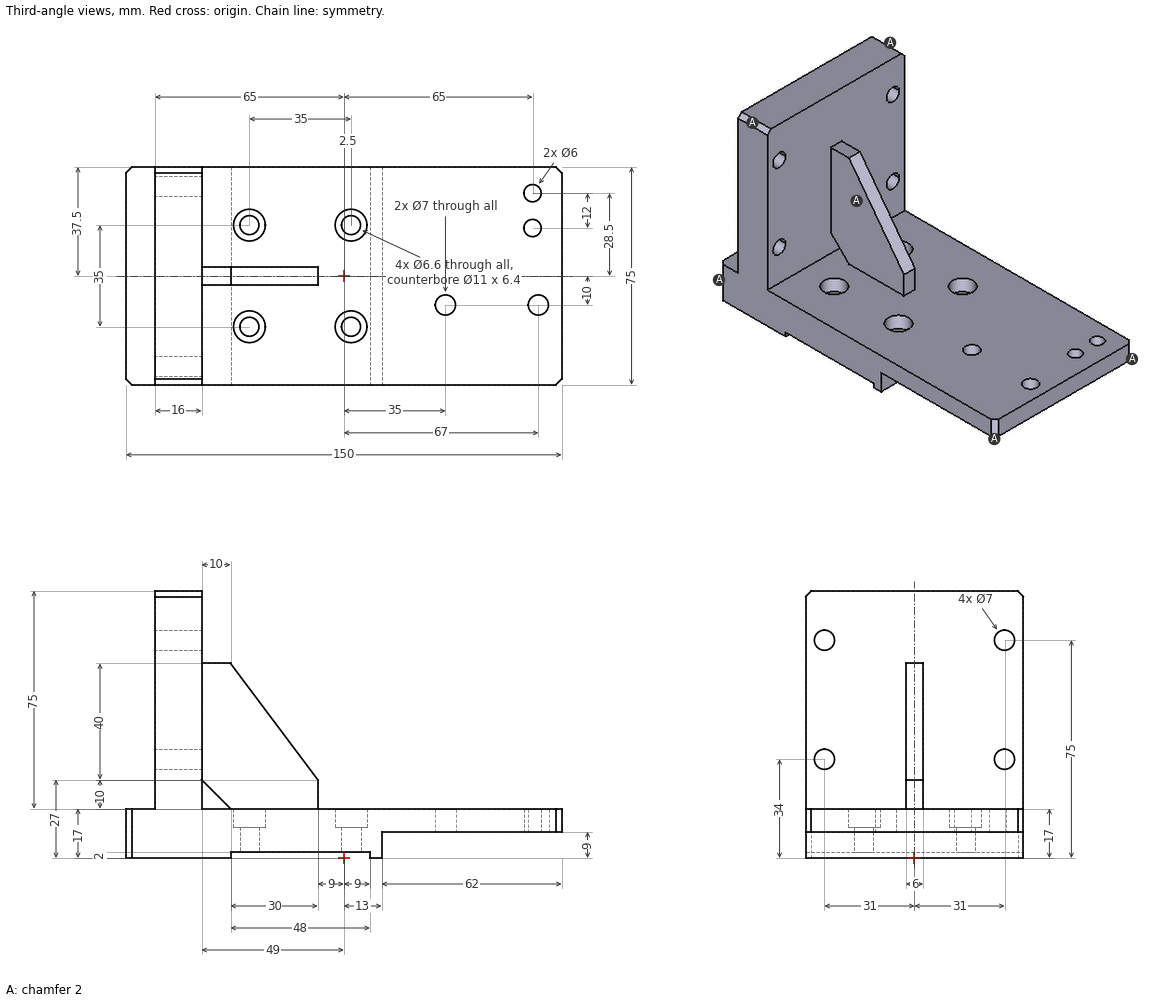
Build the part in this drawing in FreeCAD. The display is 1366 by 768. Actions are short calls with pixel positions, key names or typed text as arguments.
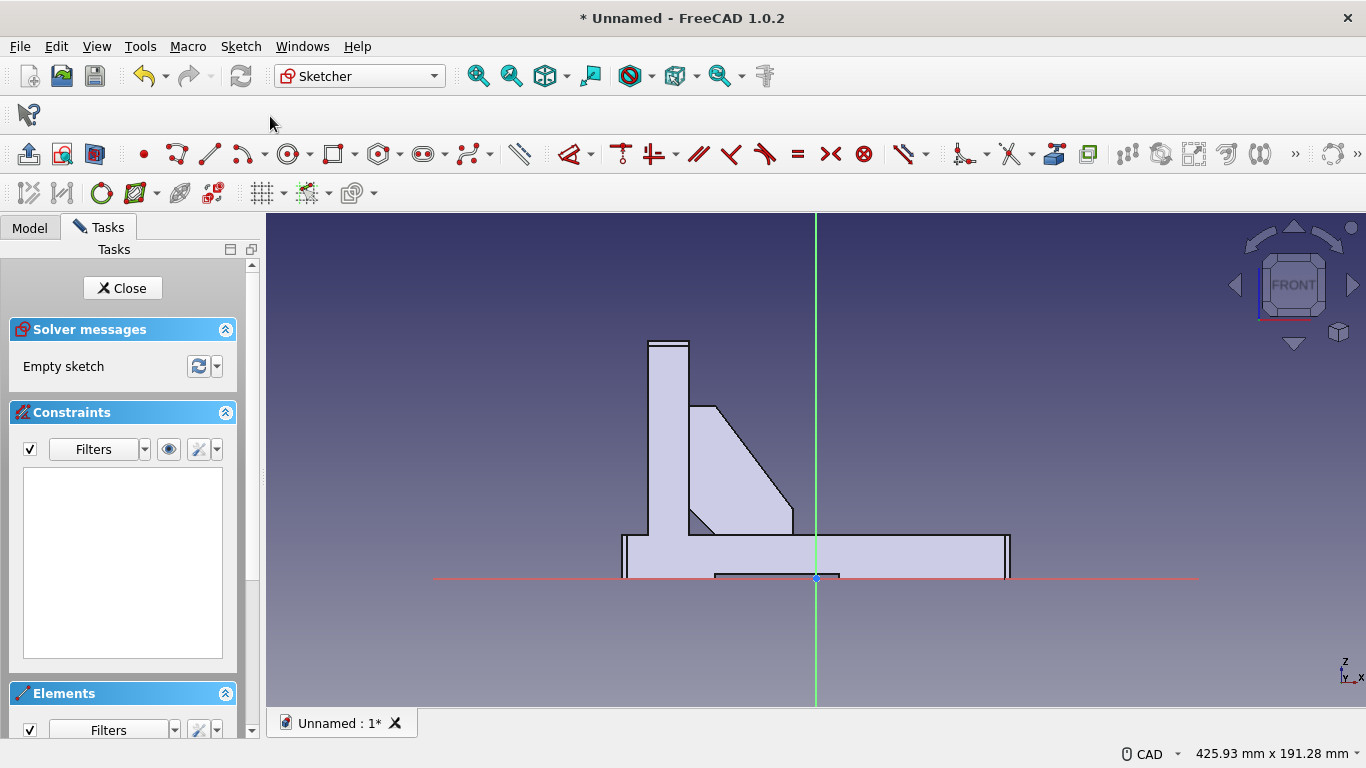
scroll(984, 613, up, 6)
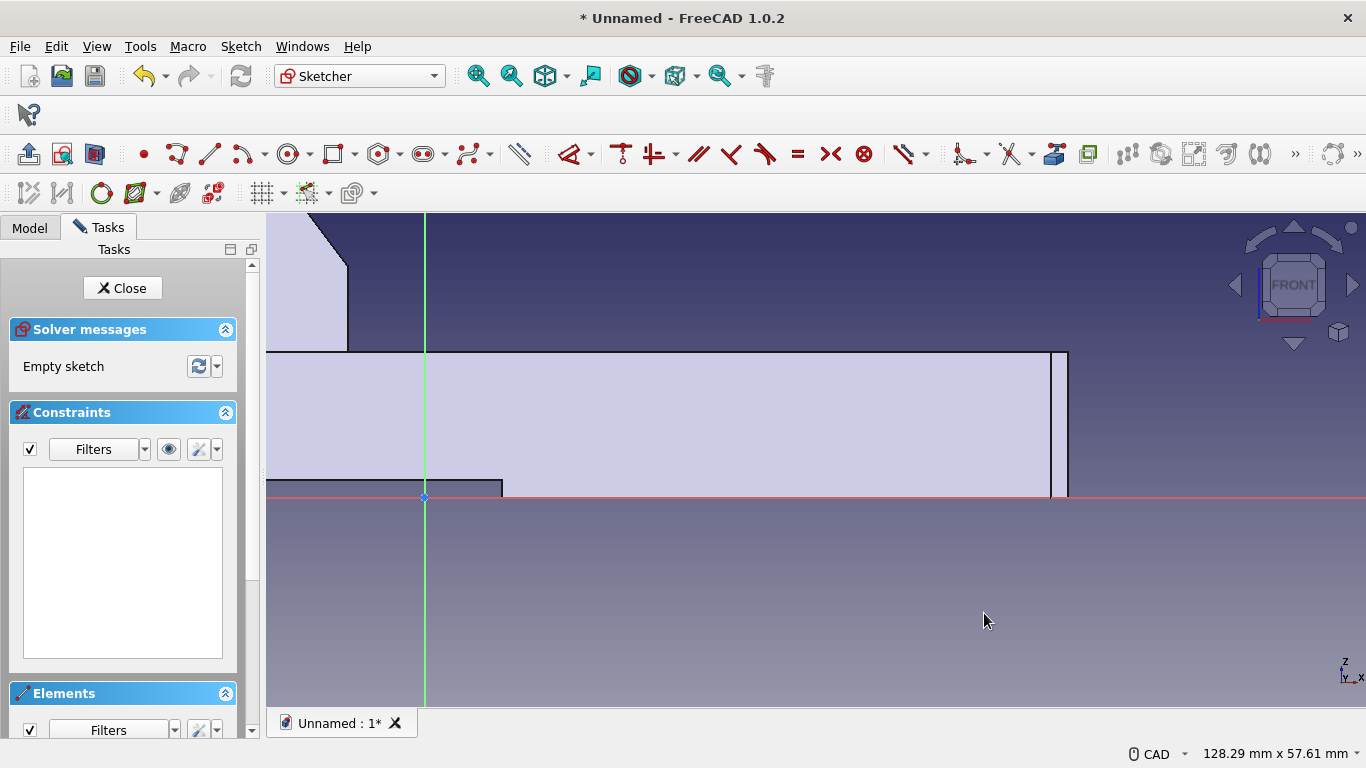
click(332, 154)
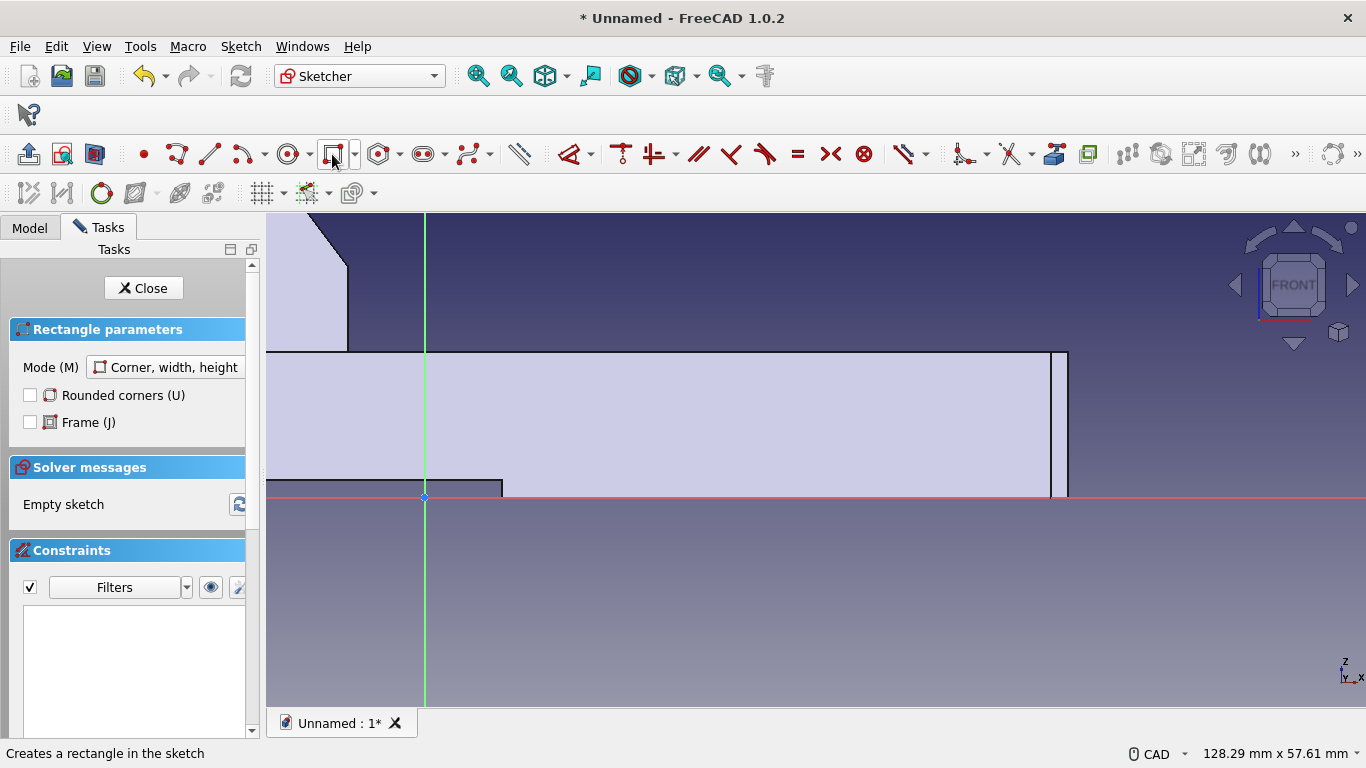
click(536, 420)
click(1068, 498)
key(Escape)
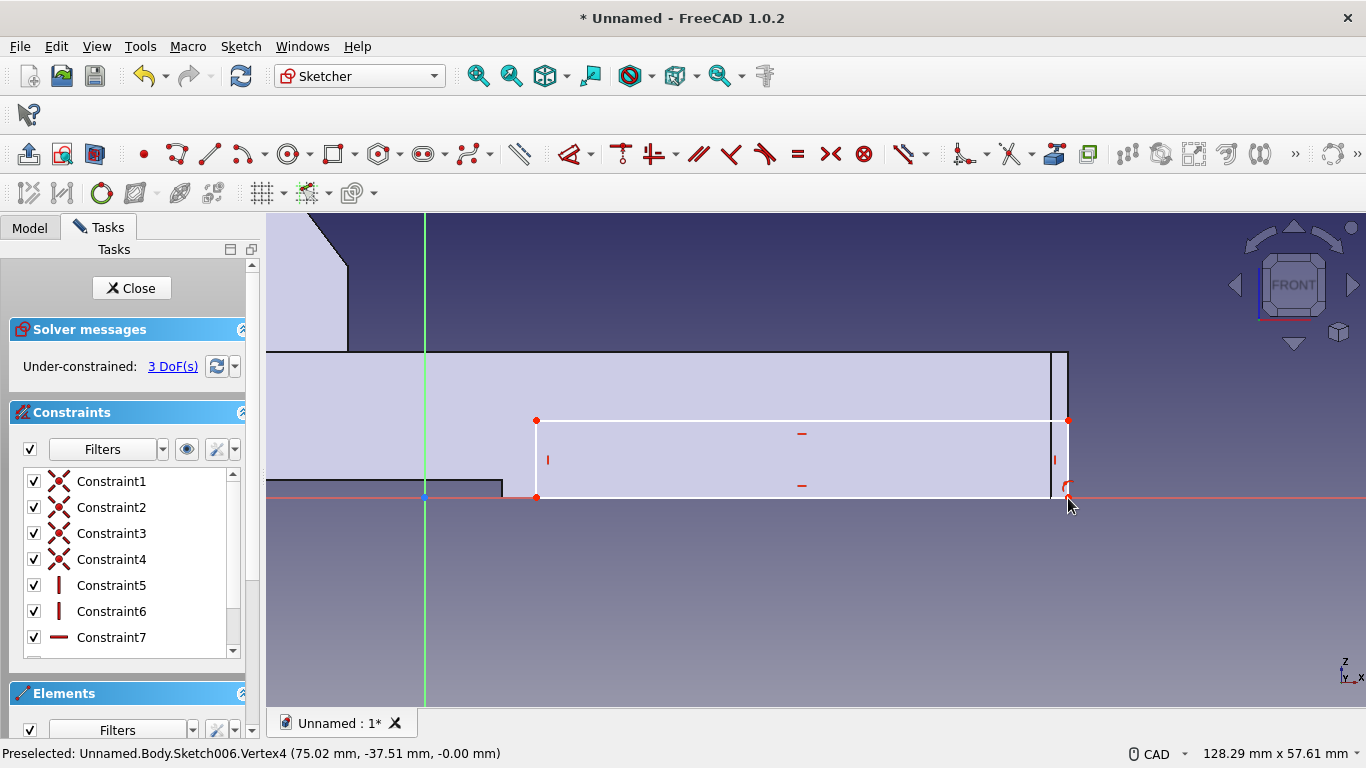
click(568, 154)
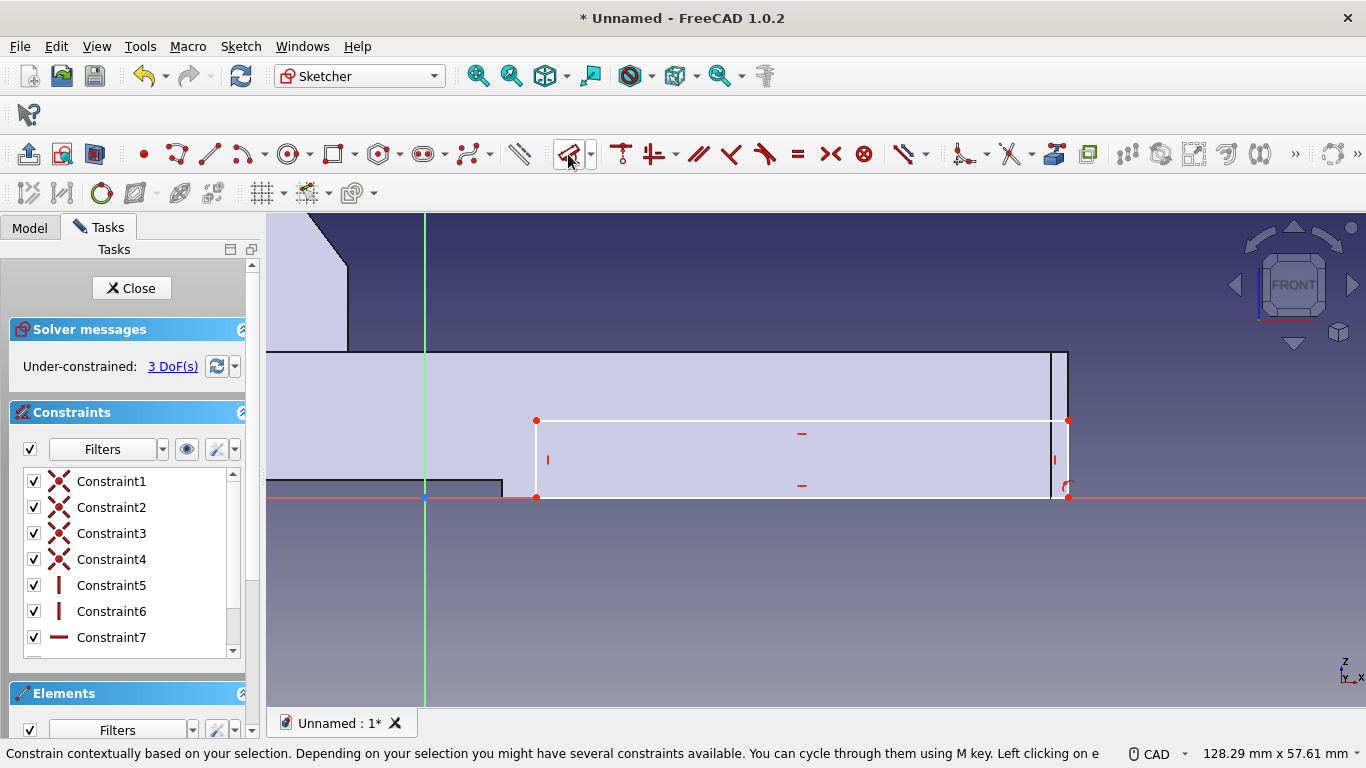
click(536, 444)
click(502, 459)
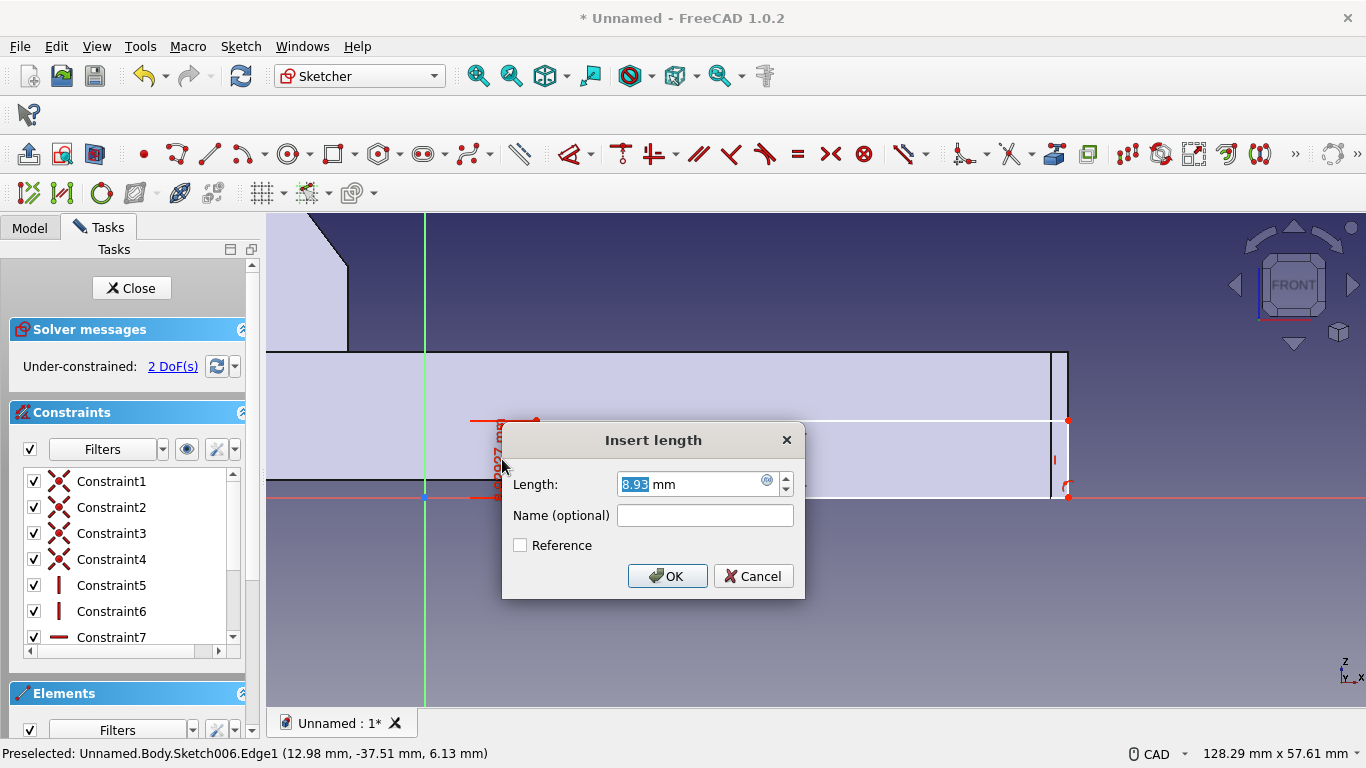
text(9)
key(Return)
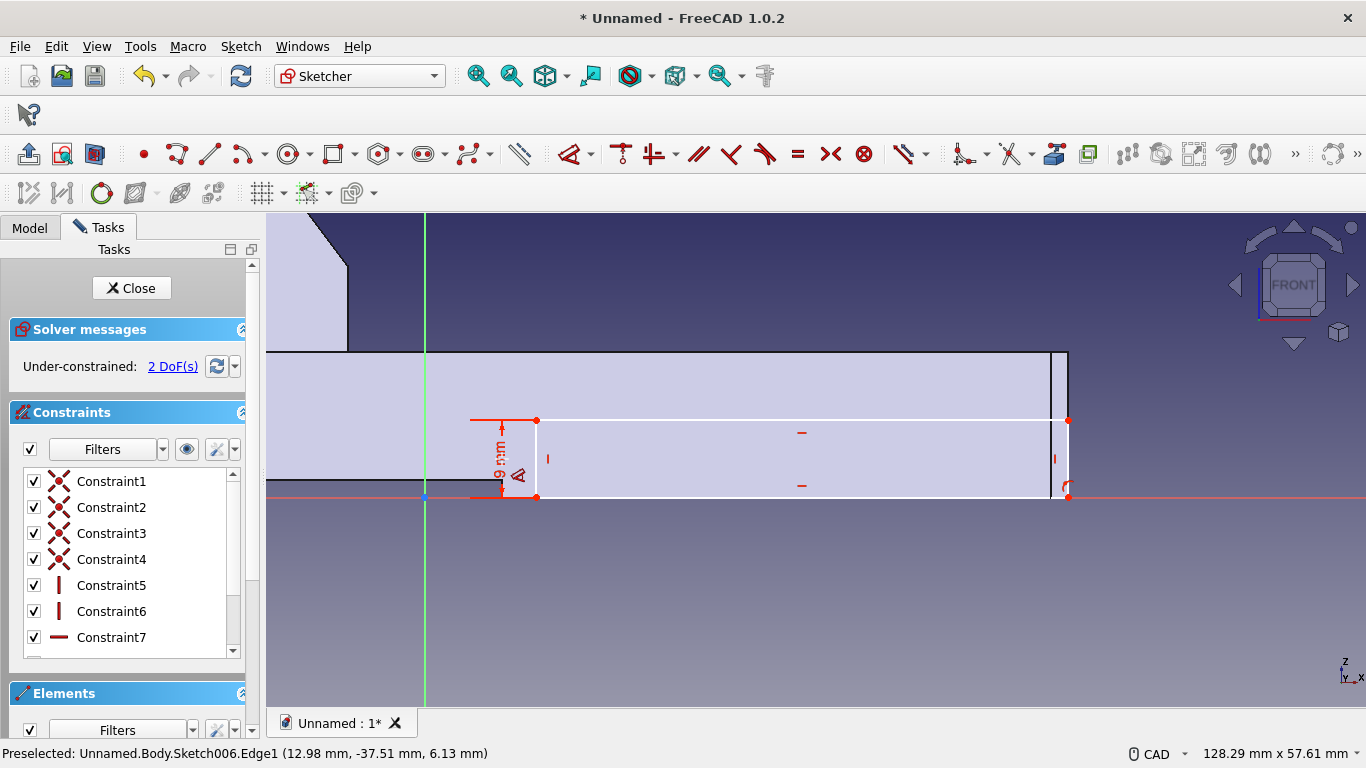
click(696, 498)
click(802, 532)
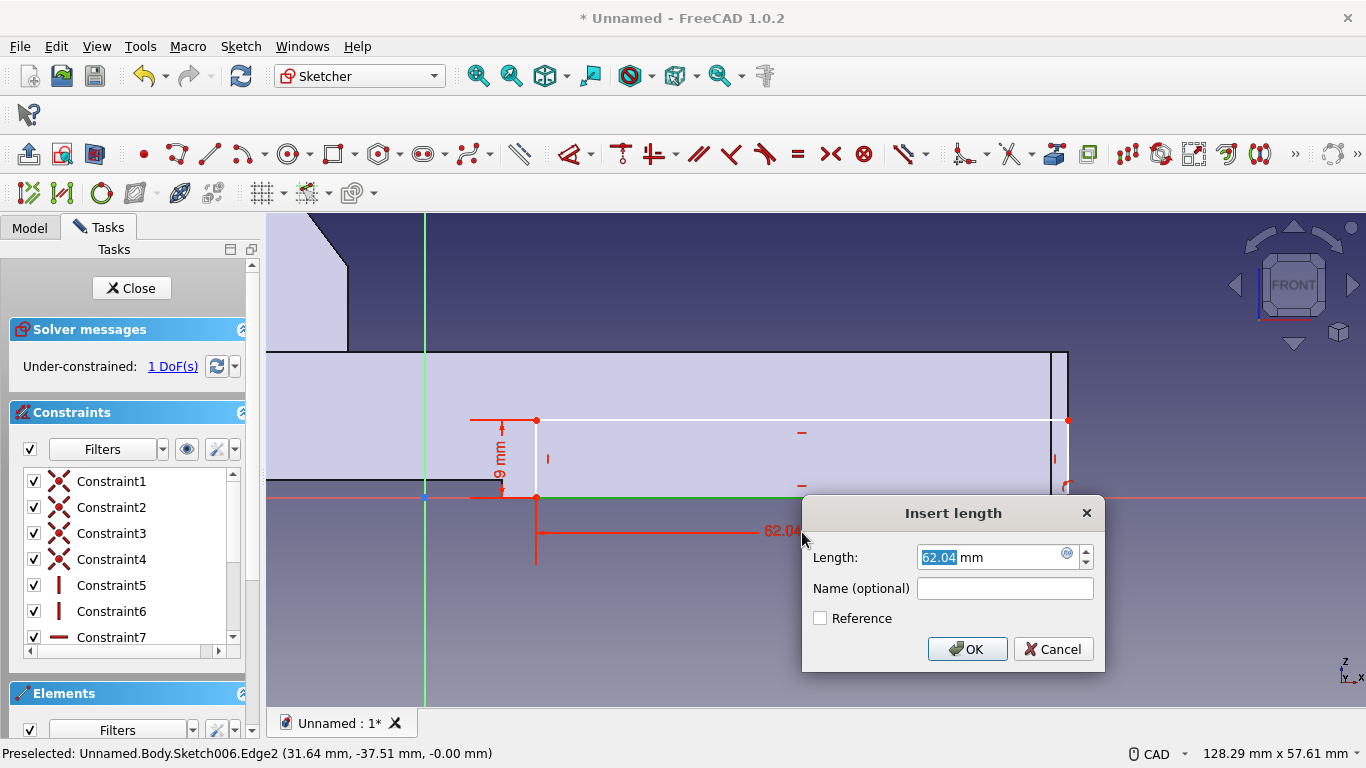
text(62)
key(Return)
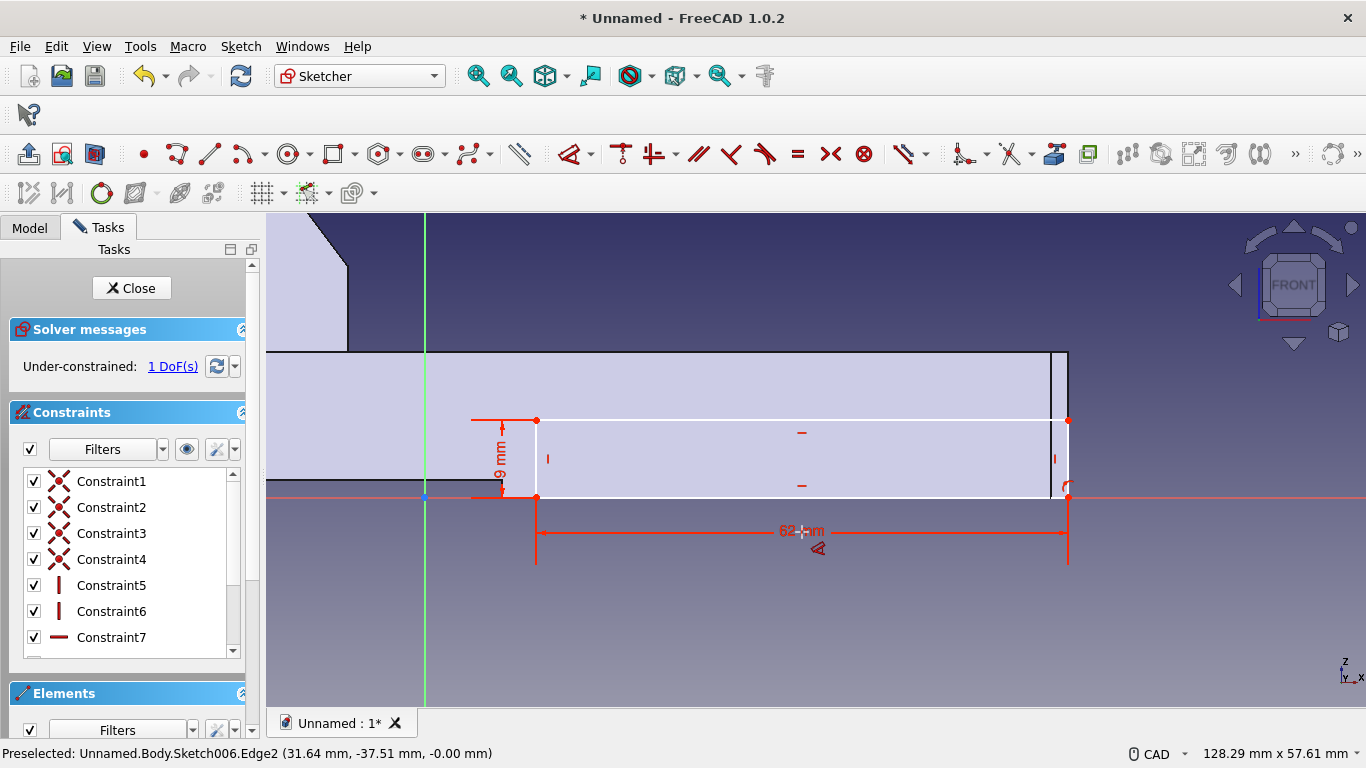
click(536, 420)
click(481, 532)